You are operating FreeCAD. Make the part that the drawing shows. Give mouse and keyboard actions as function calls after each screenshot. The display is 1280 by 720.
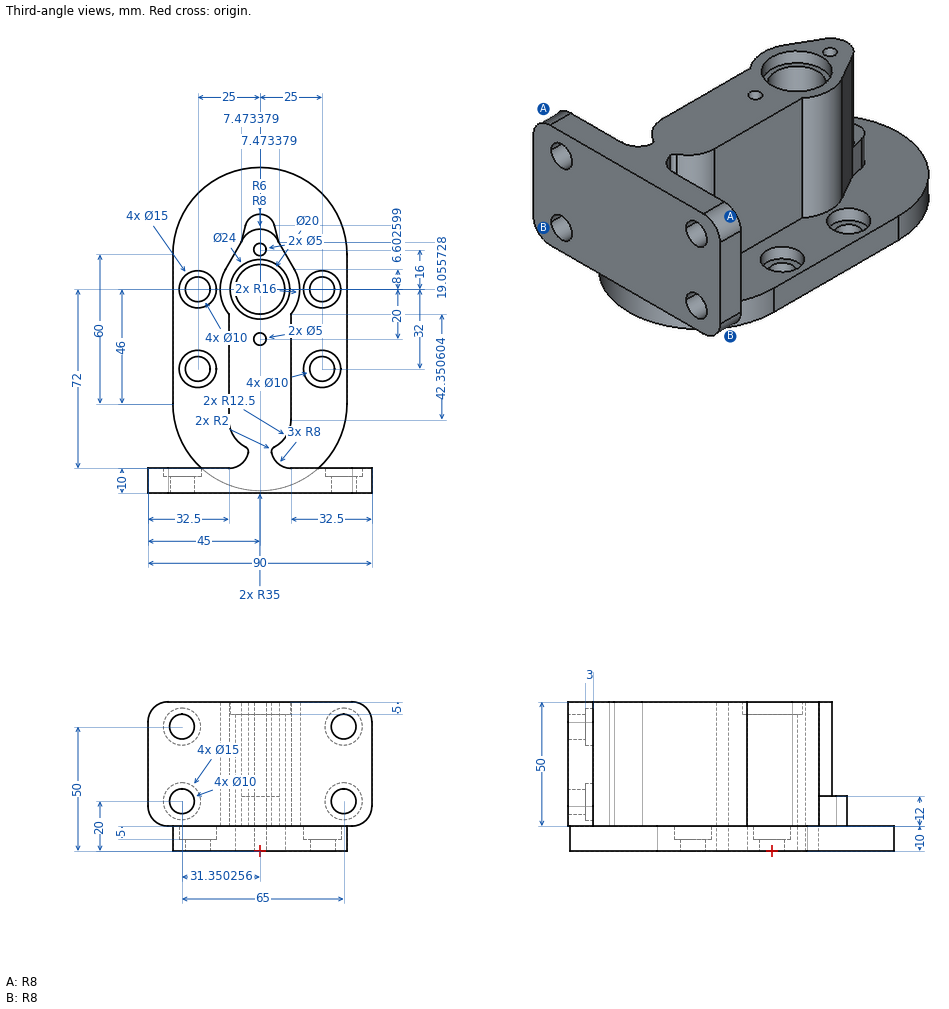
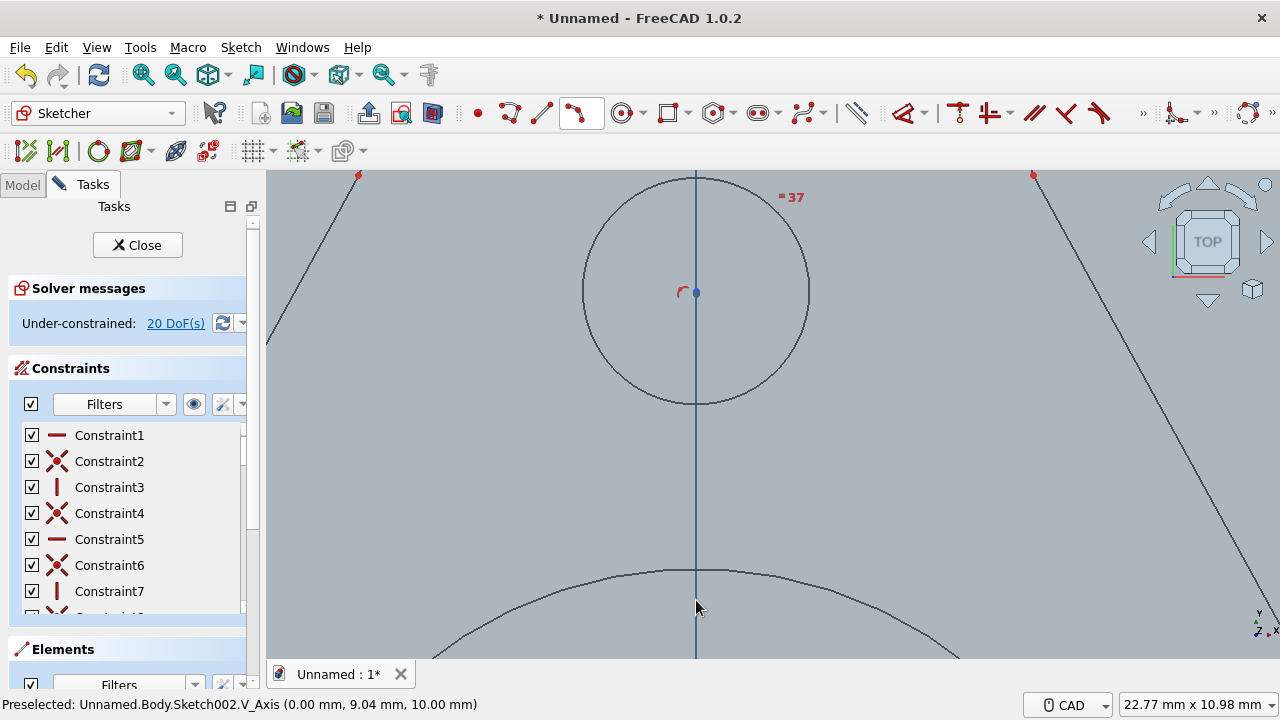
click(958, 114)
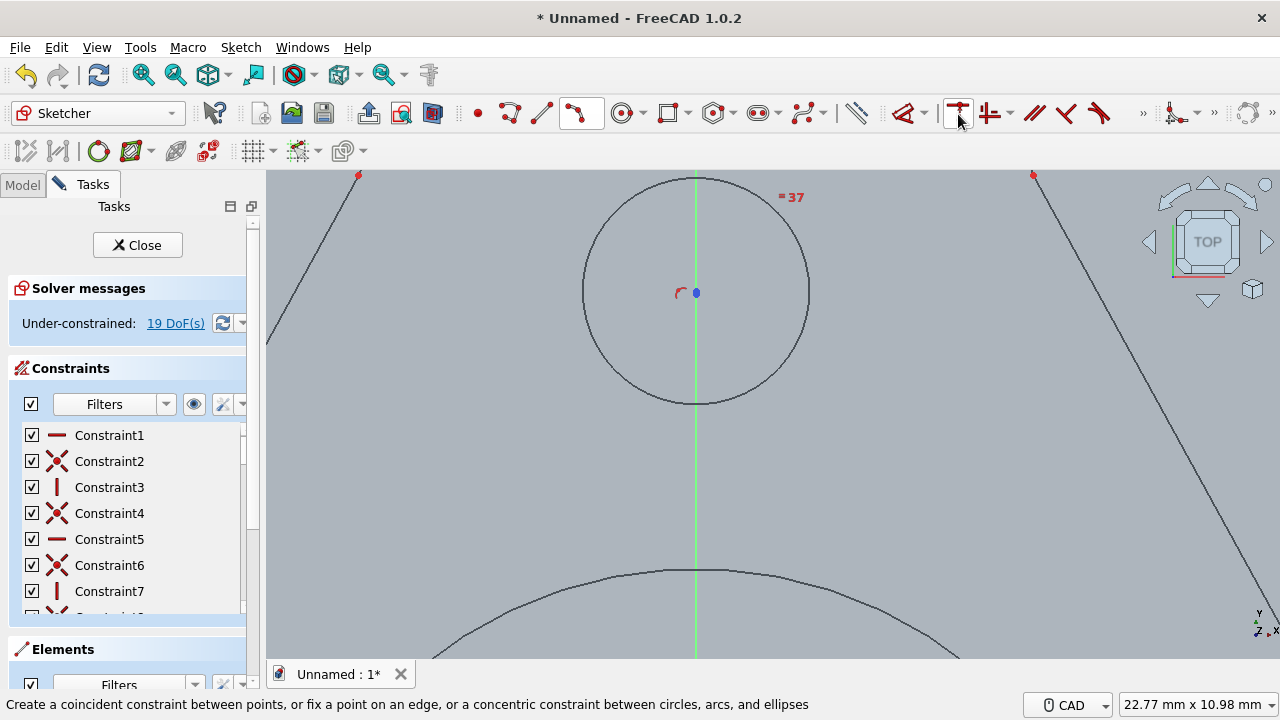
click(904, 114)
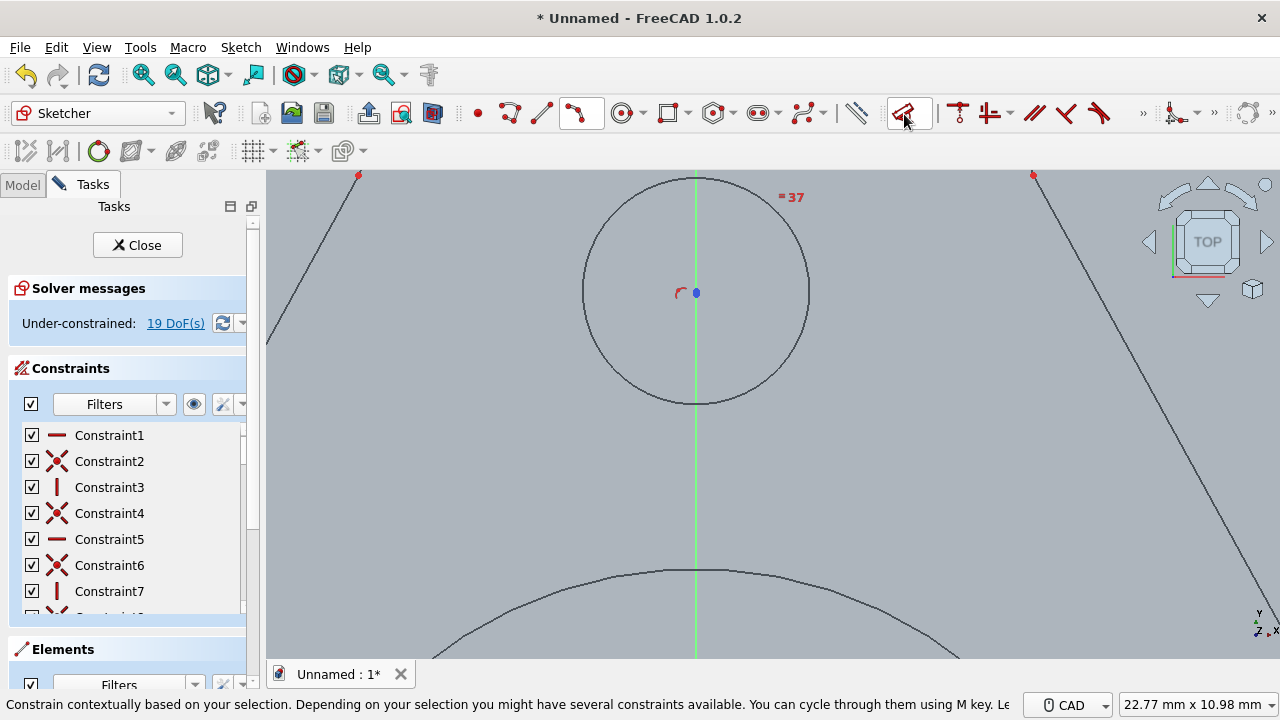
scroll(705, 293, down, 14)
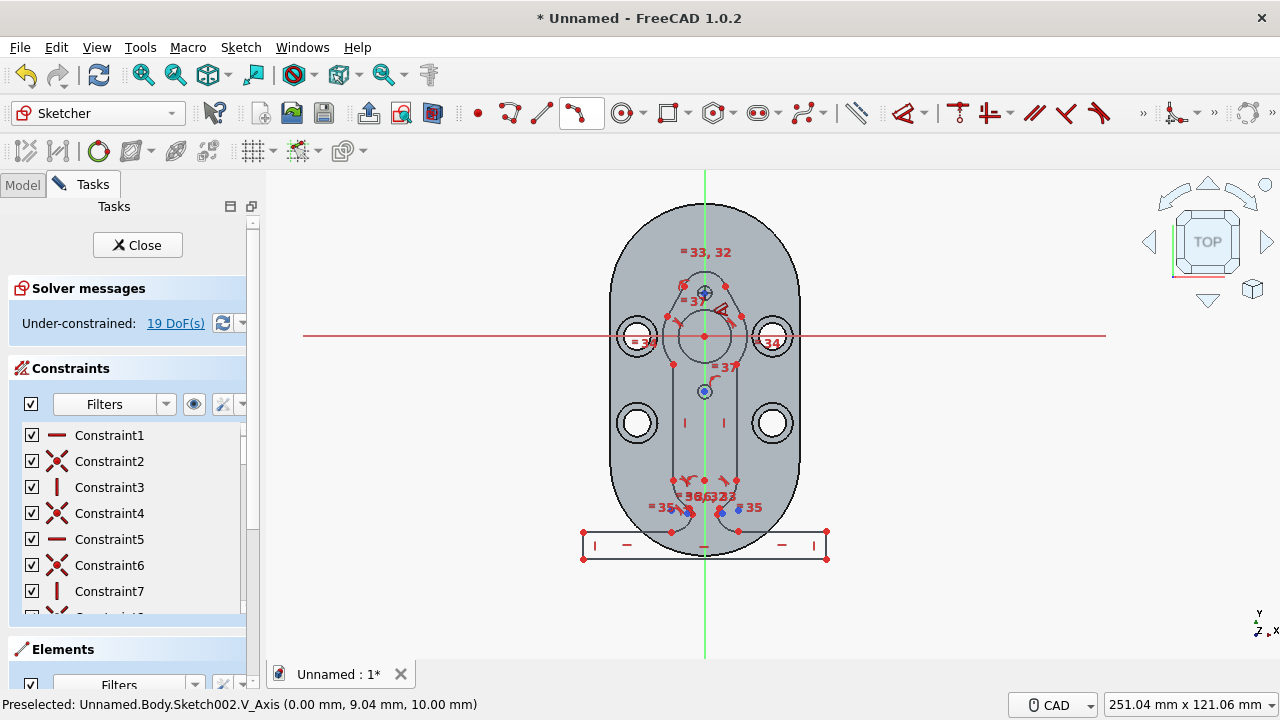
scroll(721, 523, up, 4)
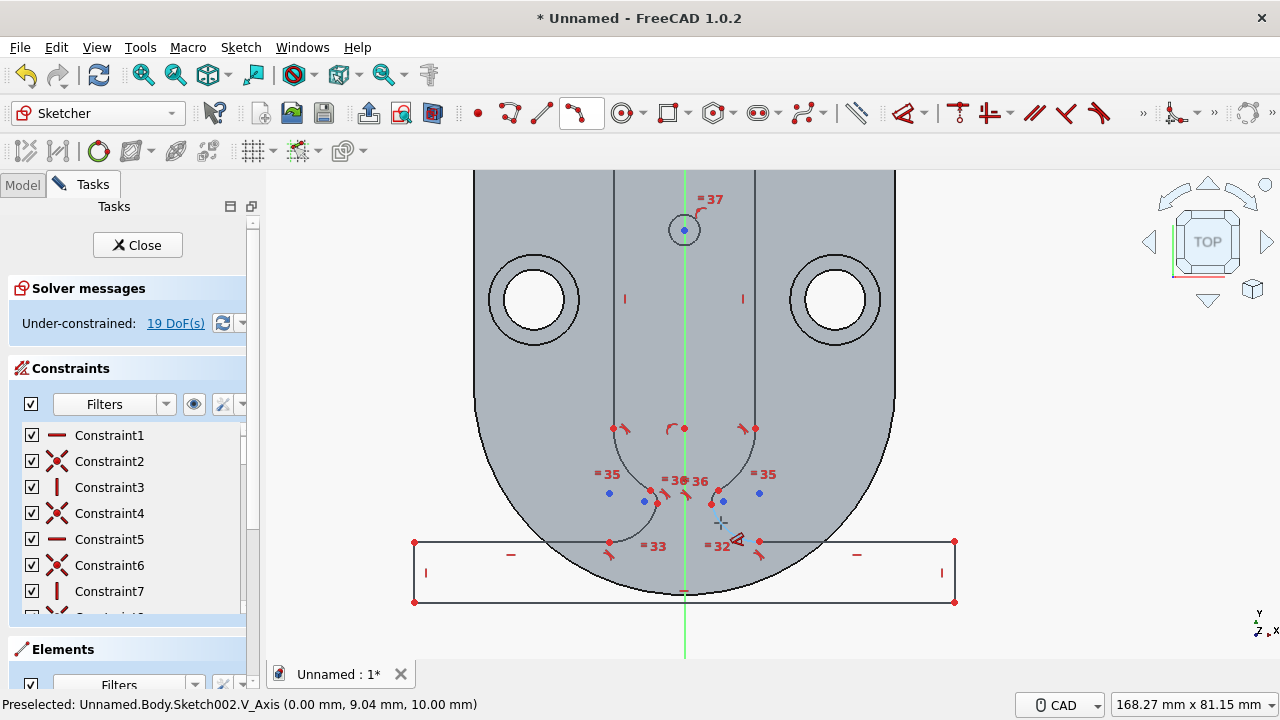
click(720, 522)
click(725, 566)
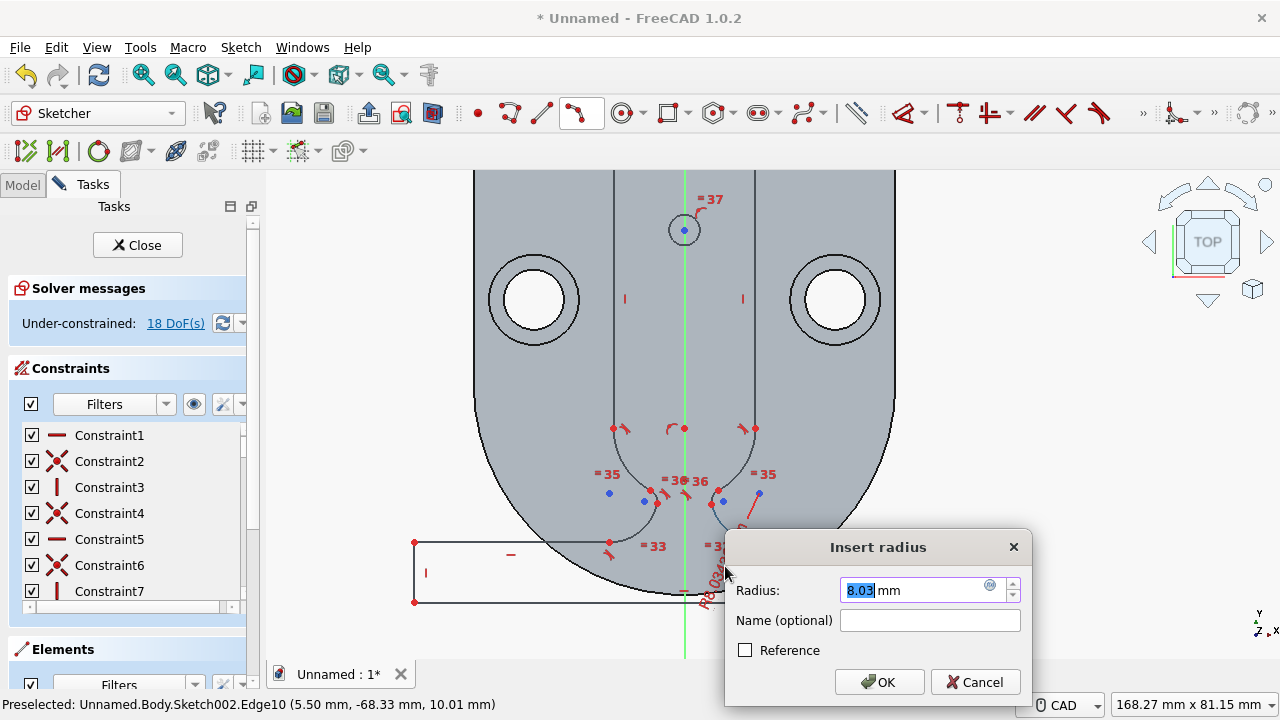
text(8)
key(Return)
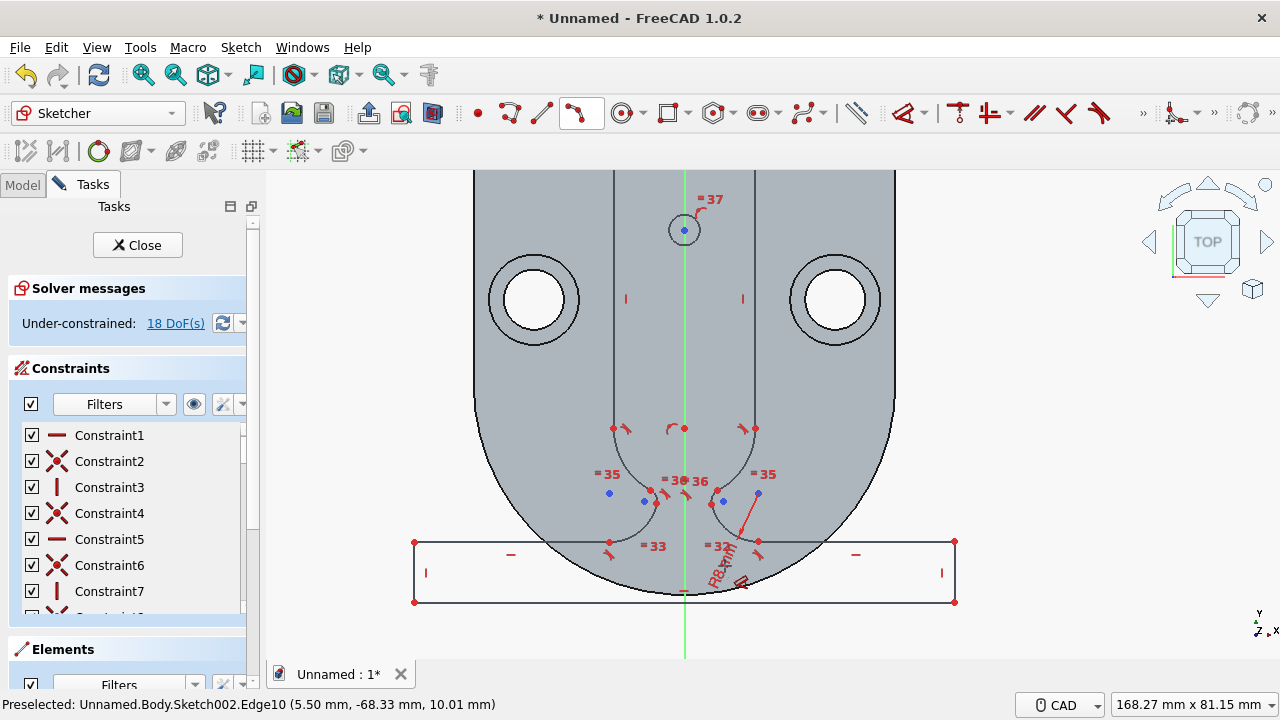
scroll(713, 496, up, 6)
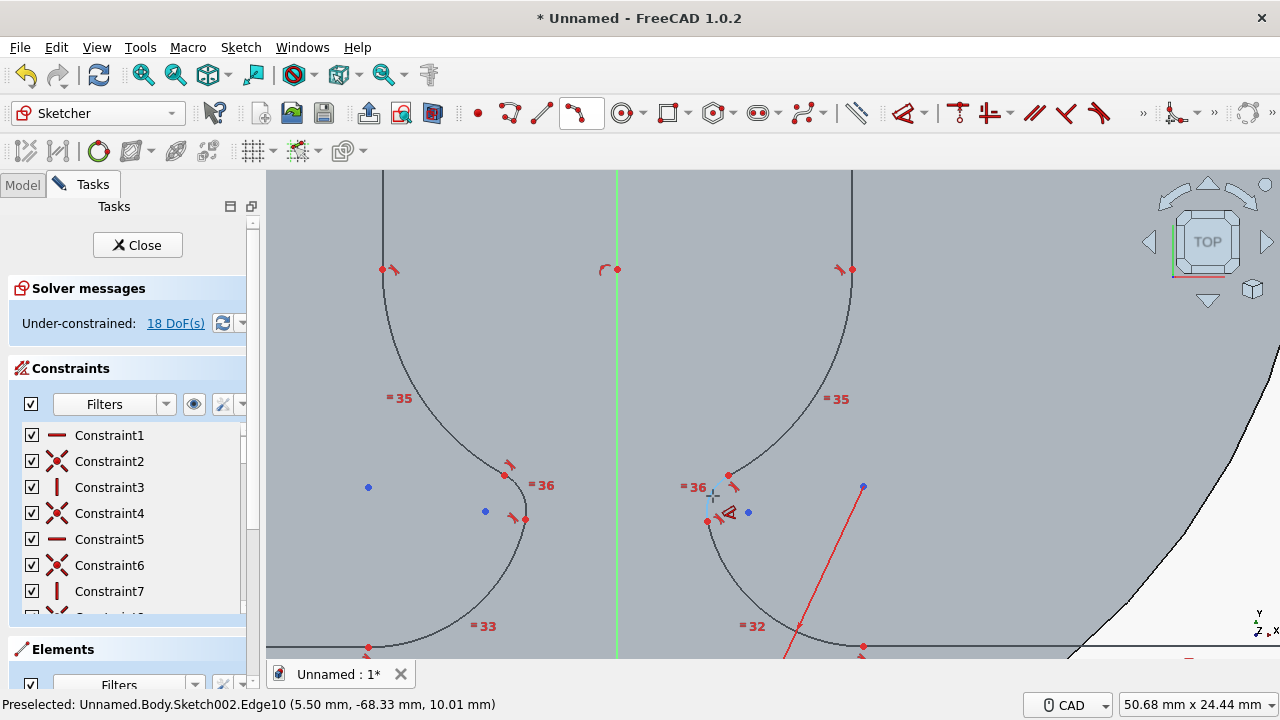
click(710, 495)
click(681, 482)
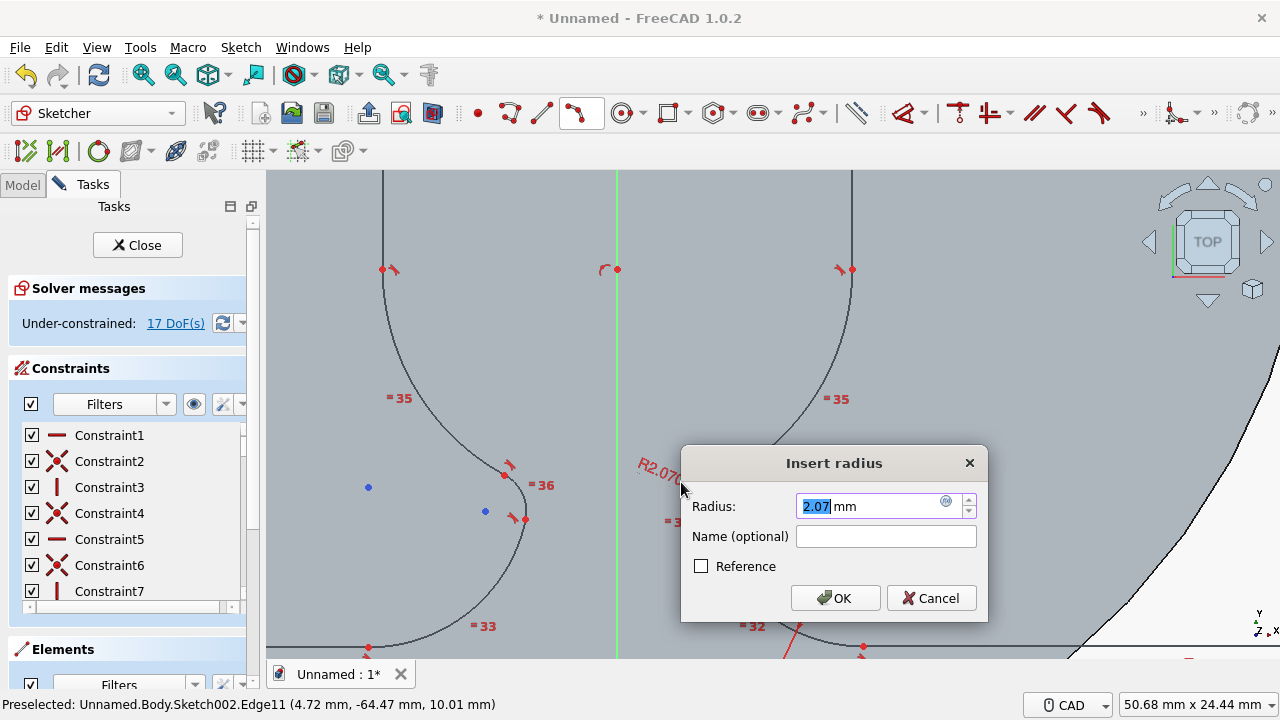
text(2)
key(Return)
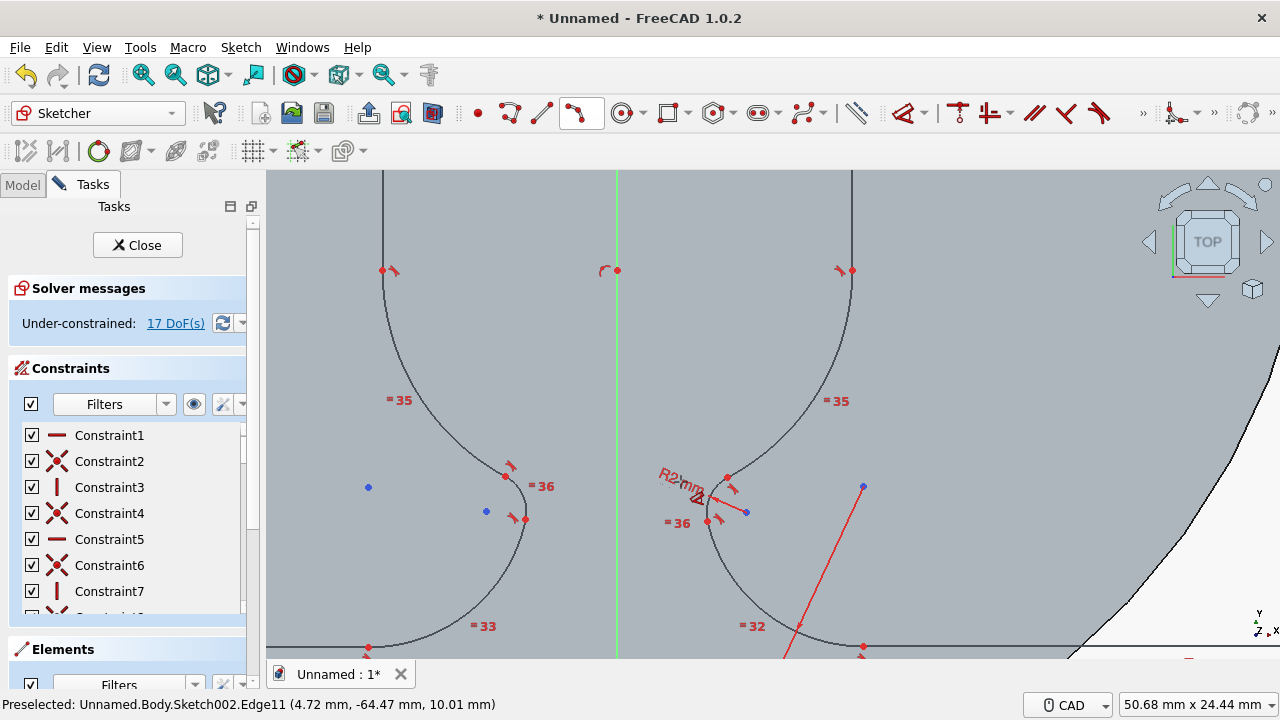
scroll(718, 514, down, 10)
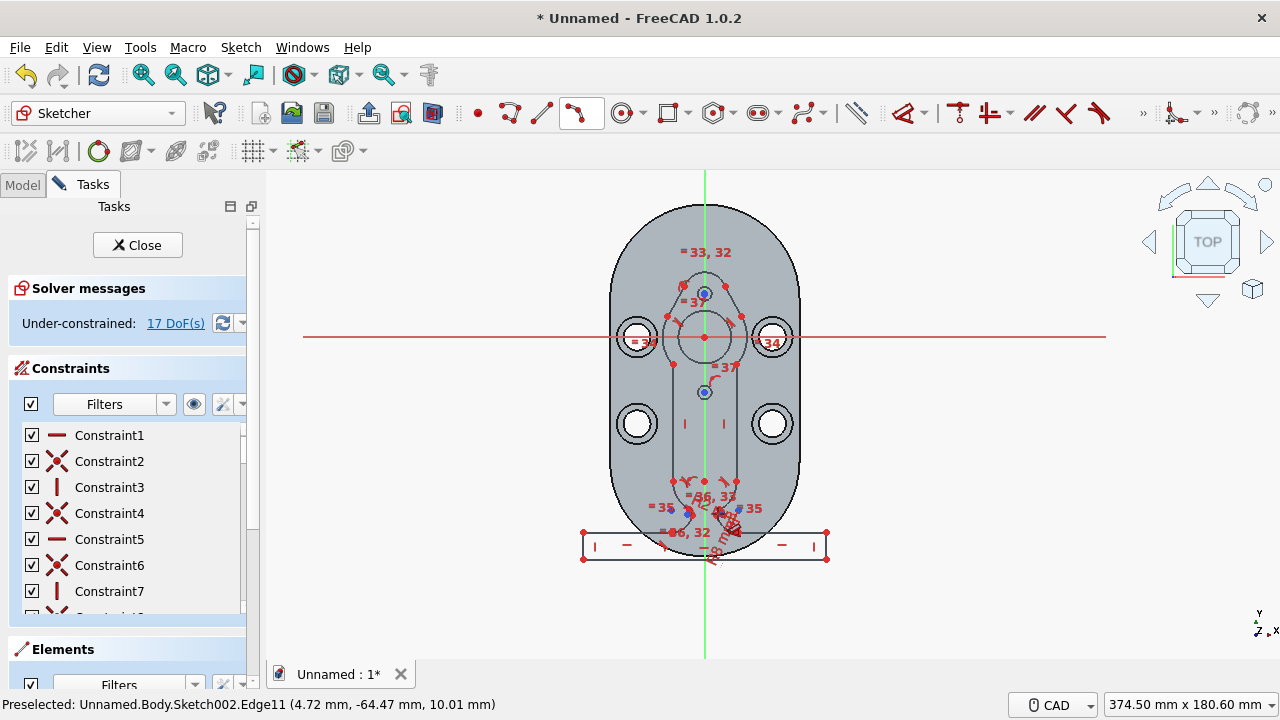
scroll(728, 503, up, 2)